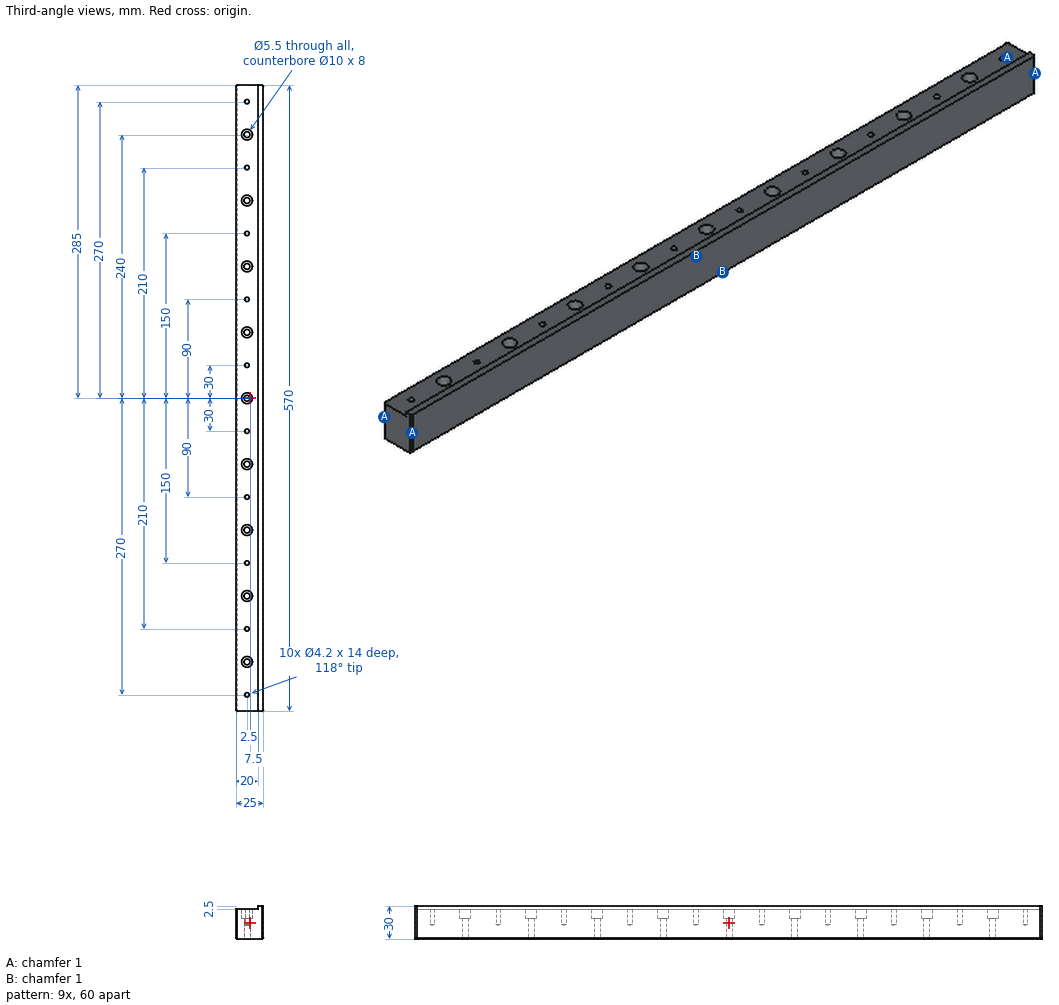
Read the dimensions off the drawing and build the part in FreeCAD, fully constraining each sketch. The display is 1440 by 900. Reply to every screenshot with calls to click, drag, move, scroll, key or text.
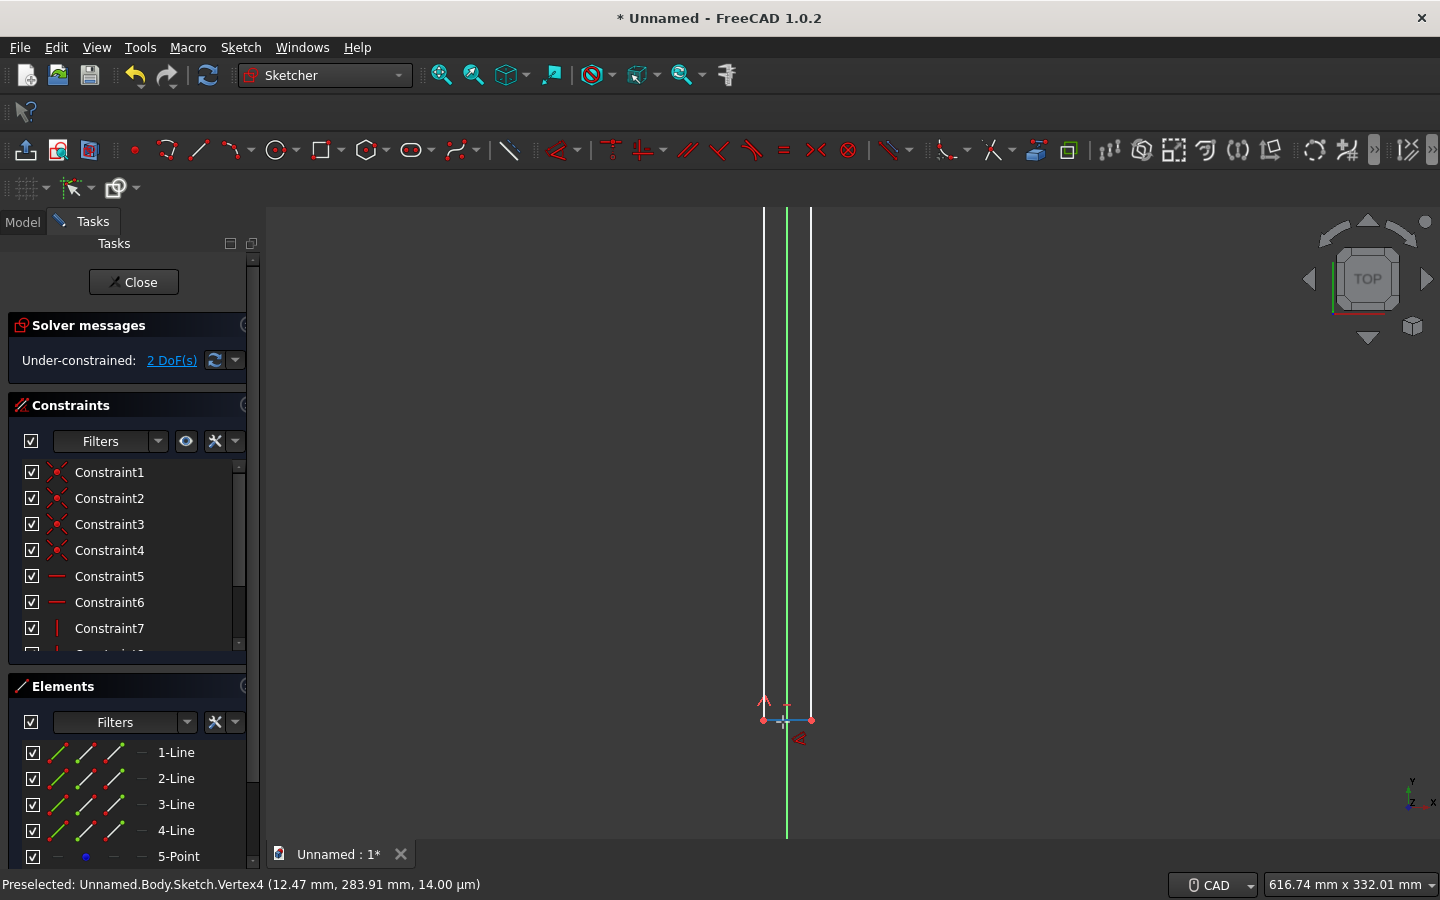
click(783, 720)
click(771, 754)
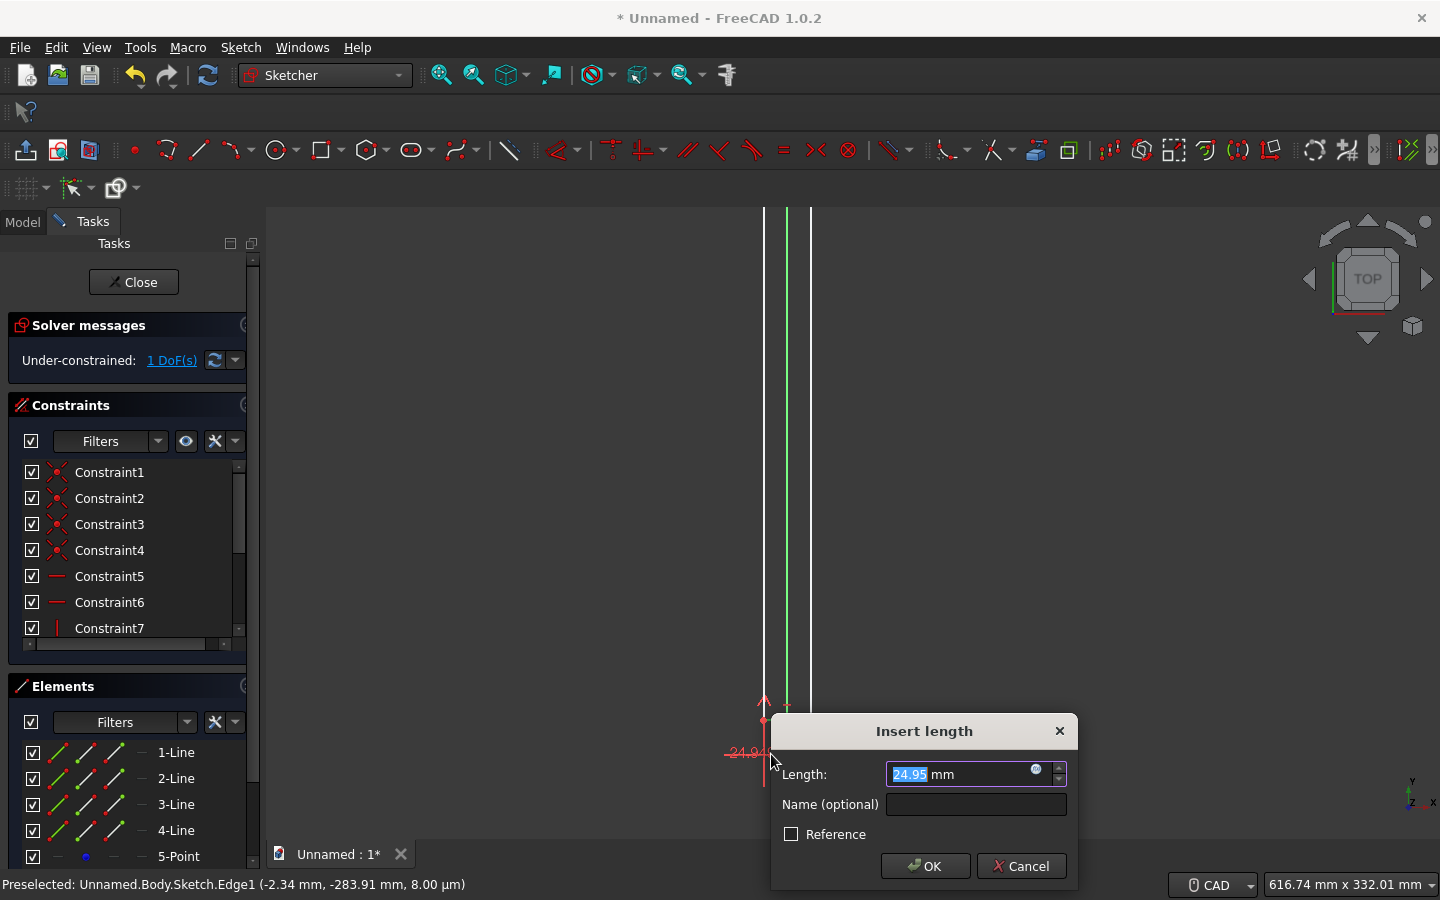
text(25)
key(Return)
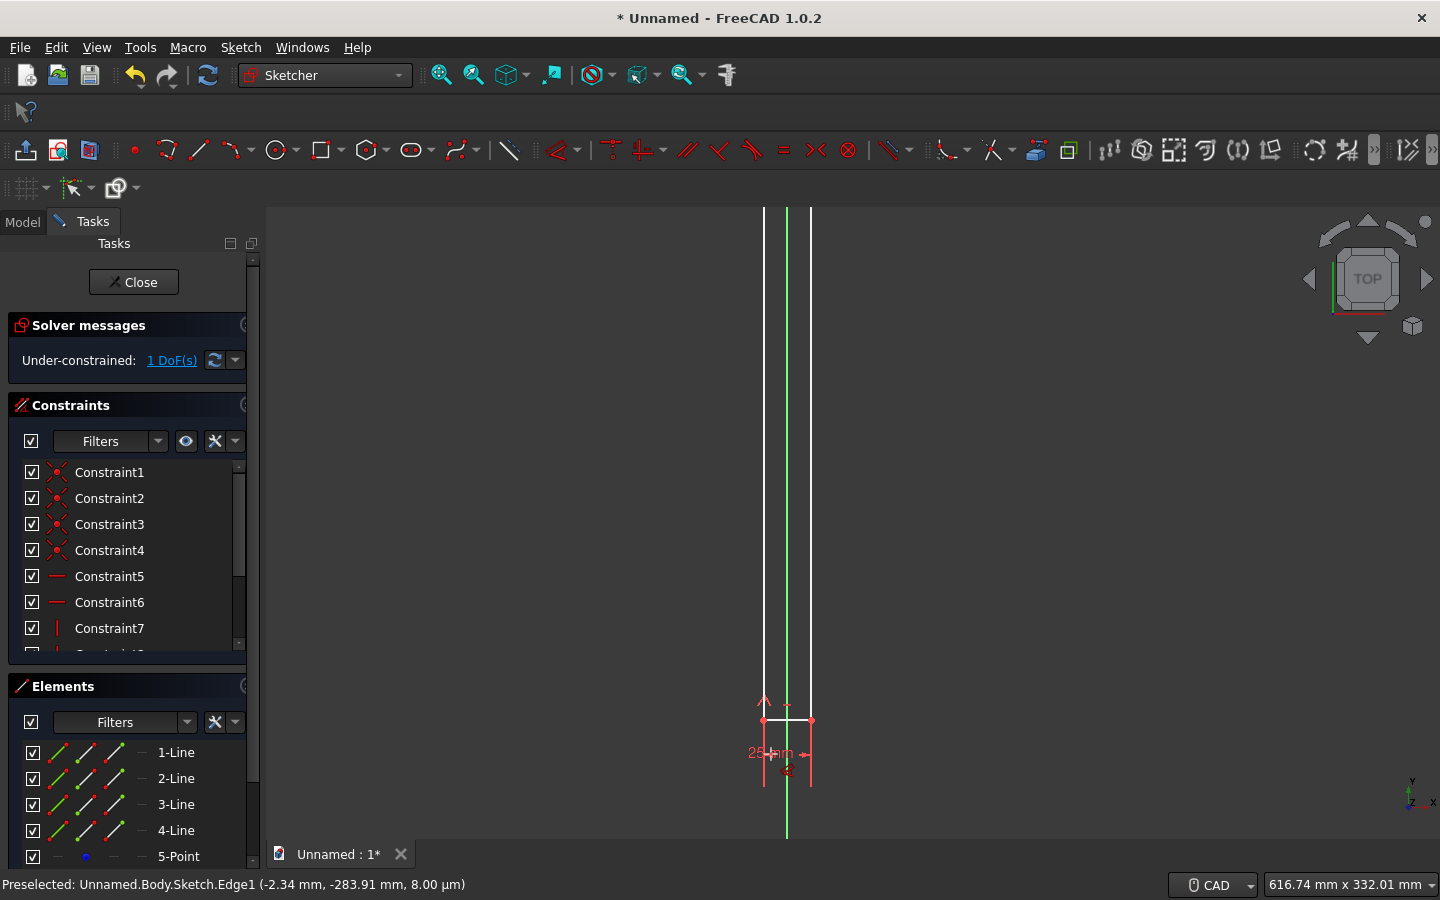
click(811, 396)
click(845, 478)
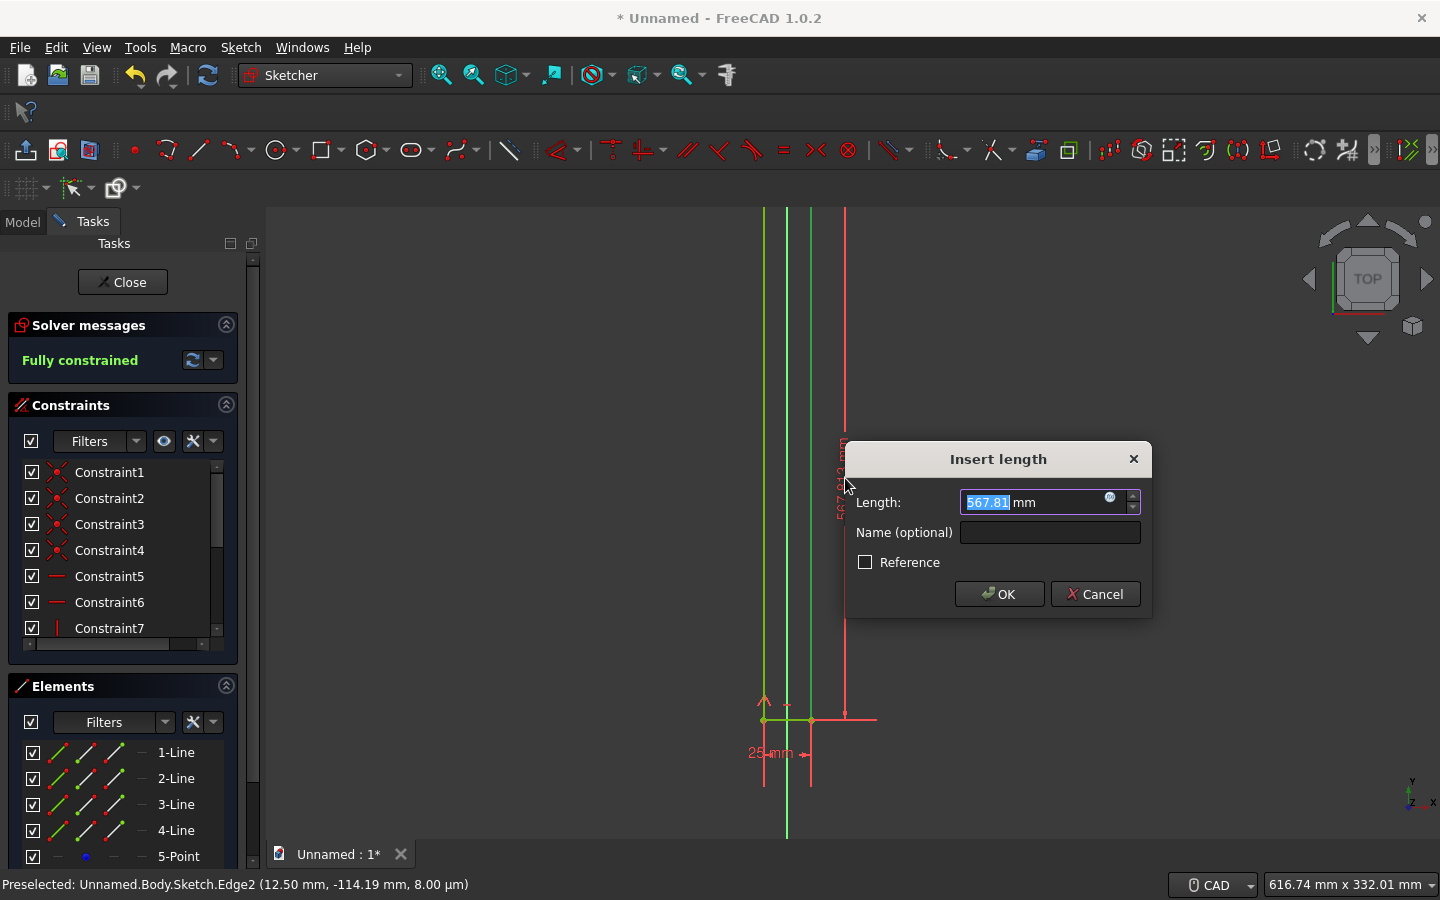
text(570)
key(Return)
key(Escape)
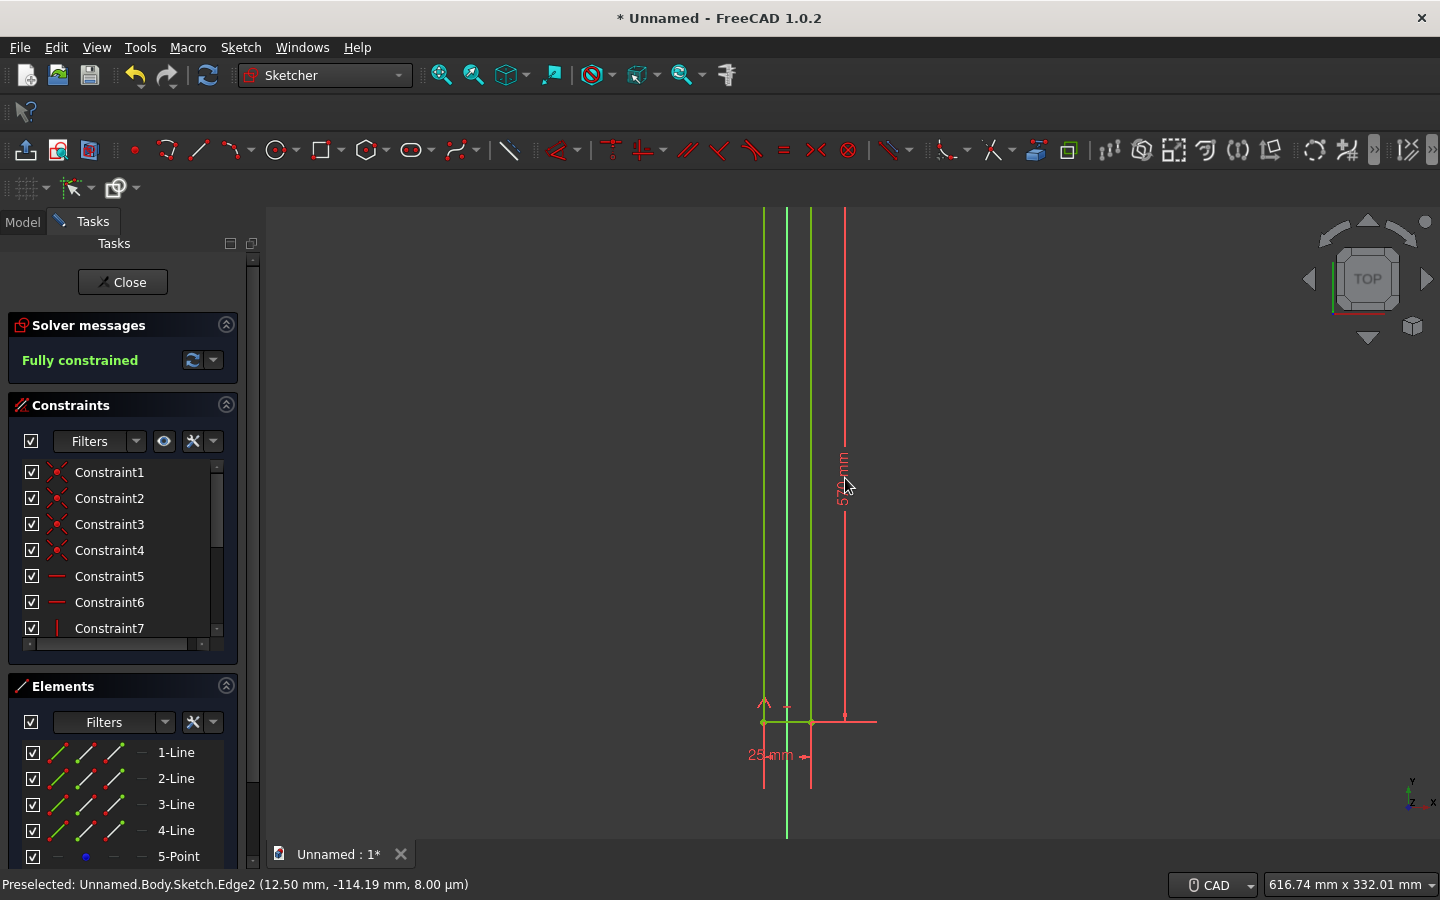
click(123, 282)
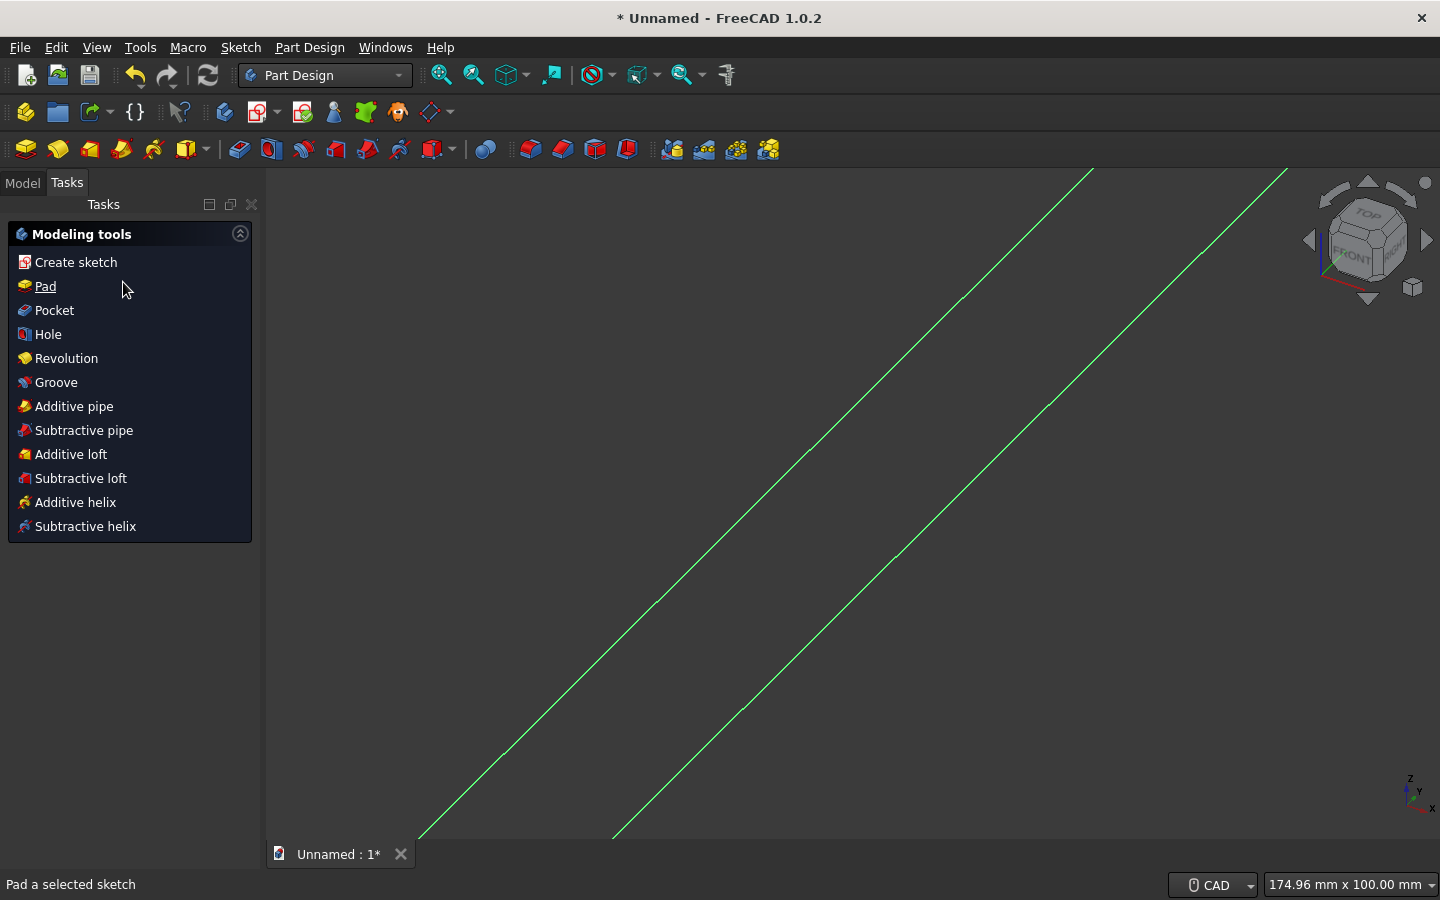
click(26, 150)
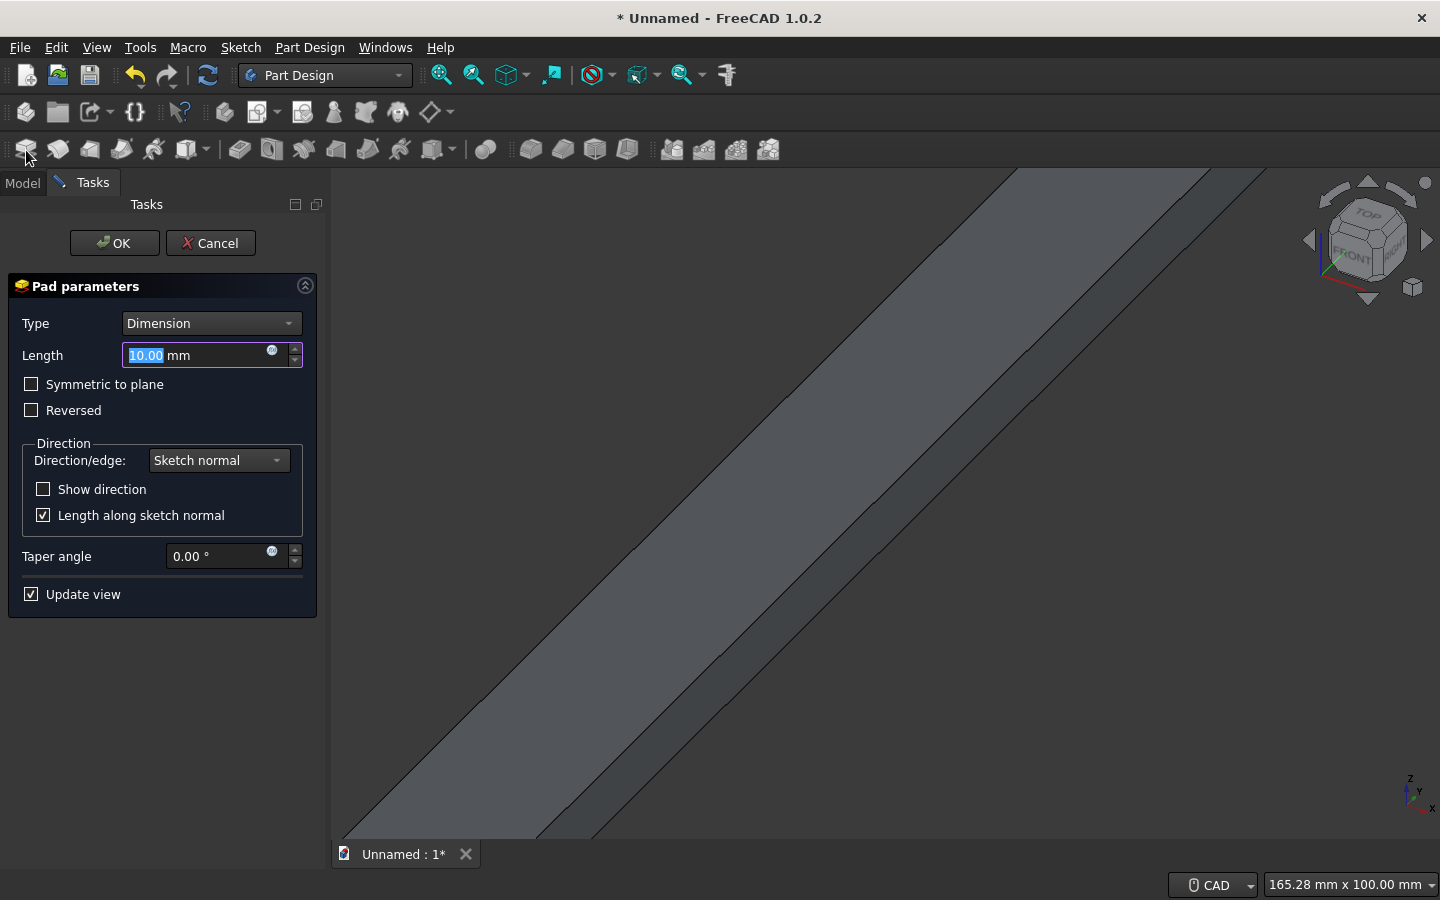
text(30)
key(Tab)